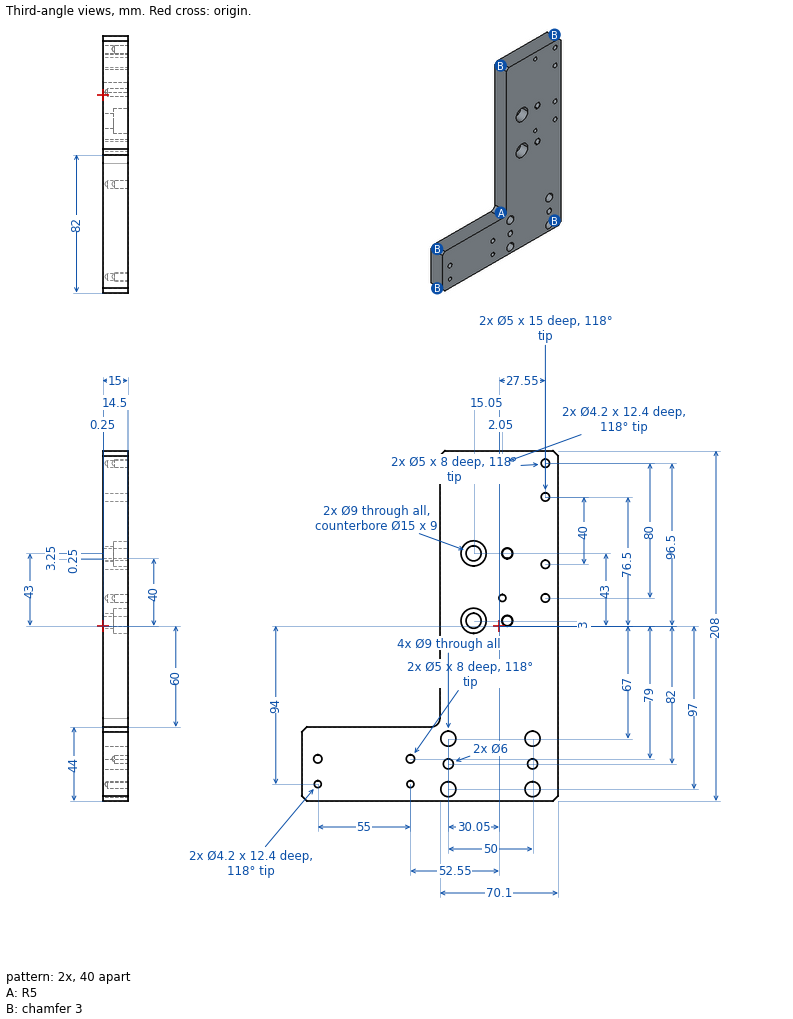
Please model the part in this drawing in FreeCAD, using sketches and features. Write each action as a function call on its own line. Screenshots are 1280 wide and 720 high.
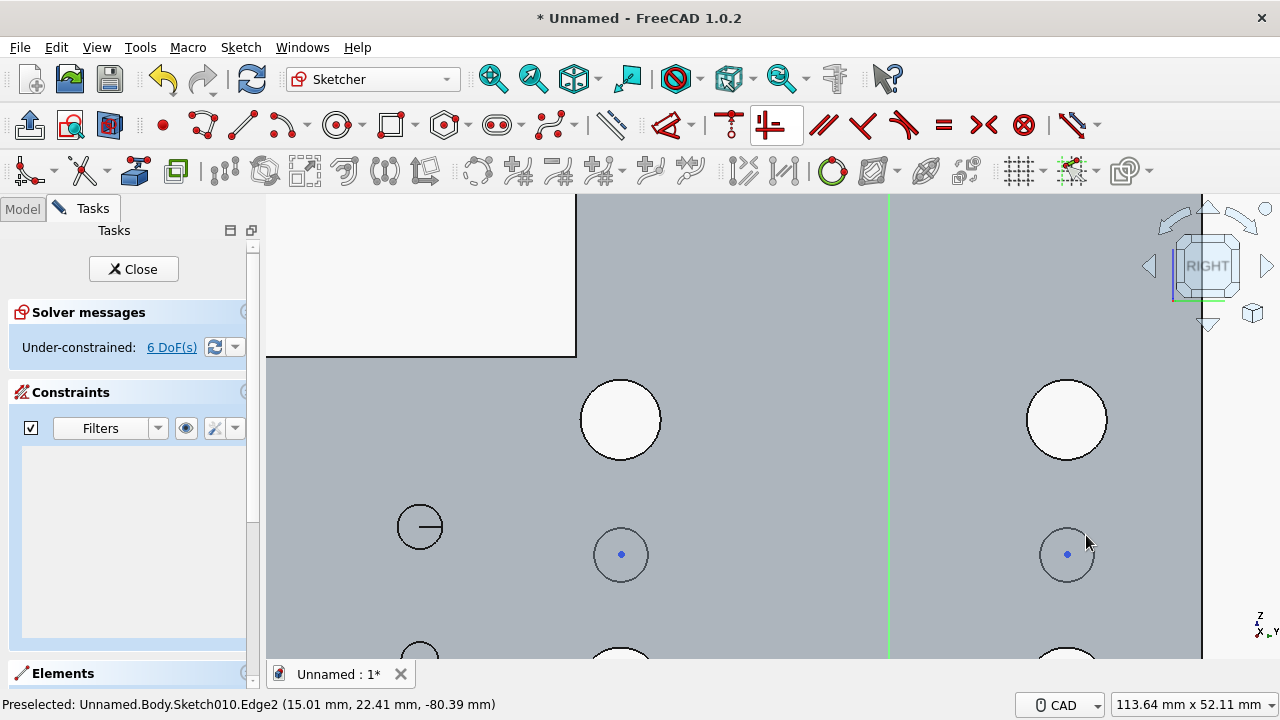
click(640, 536)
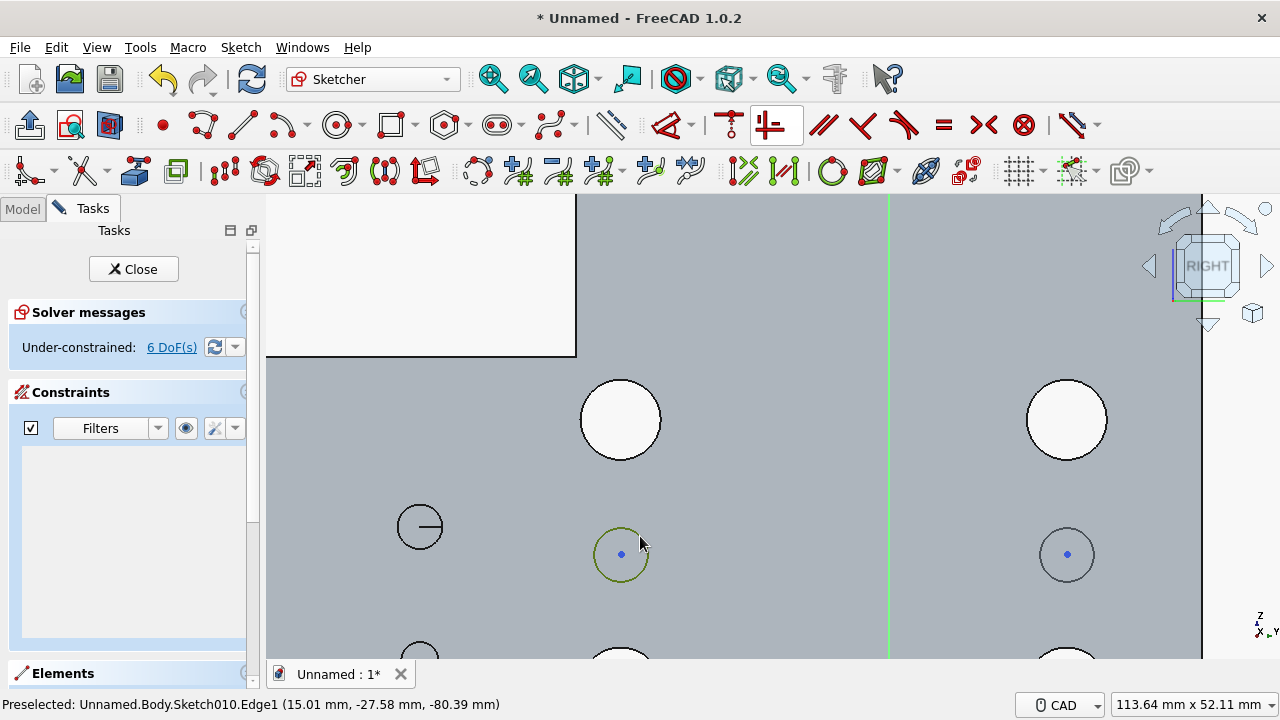
click(1086, 536)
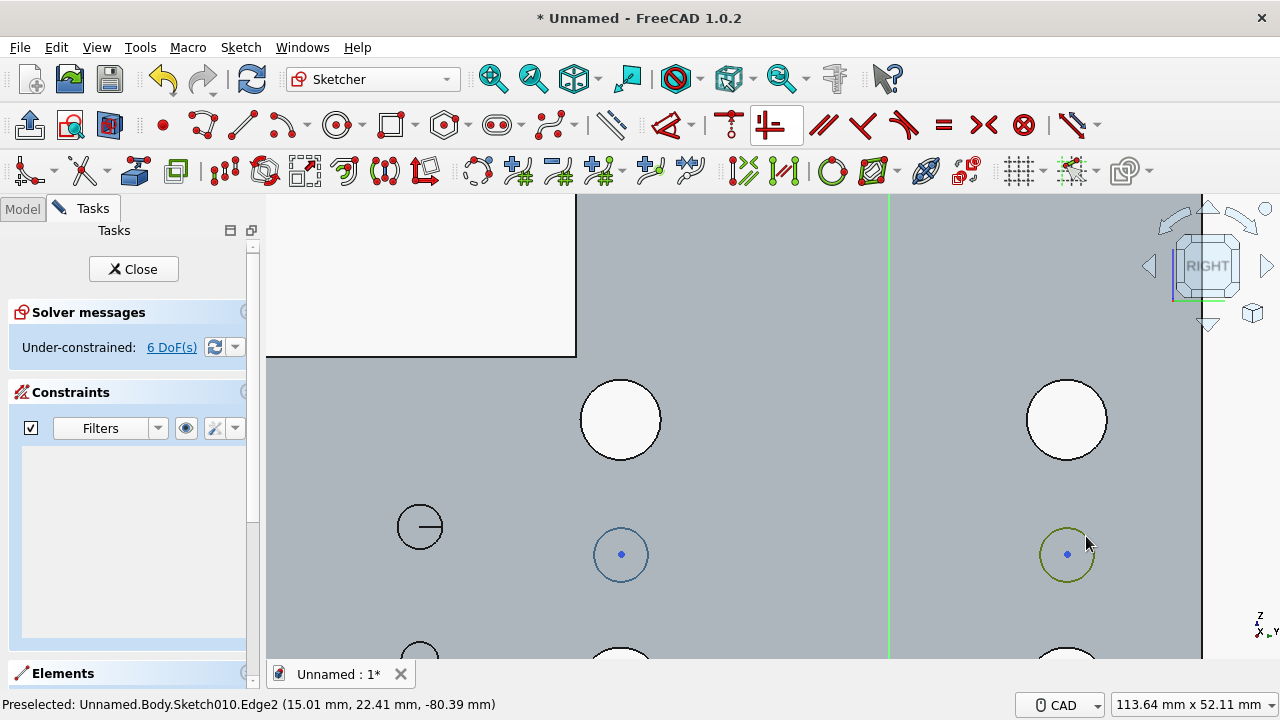
click(944, 126)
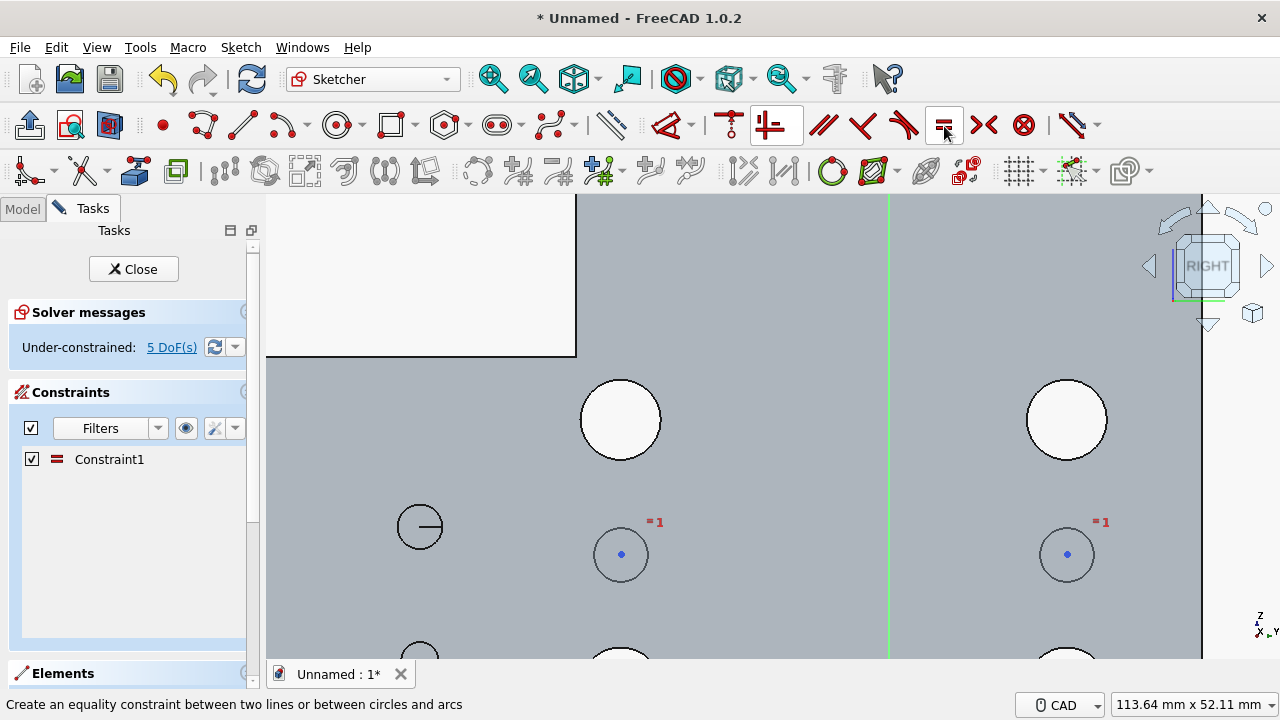
click(621, 555)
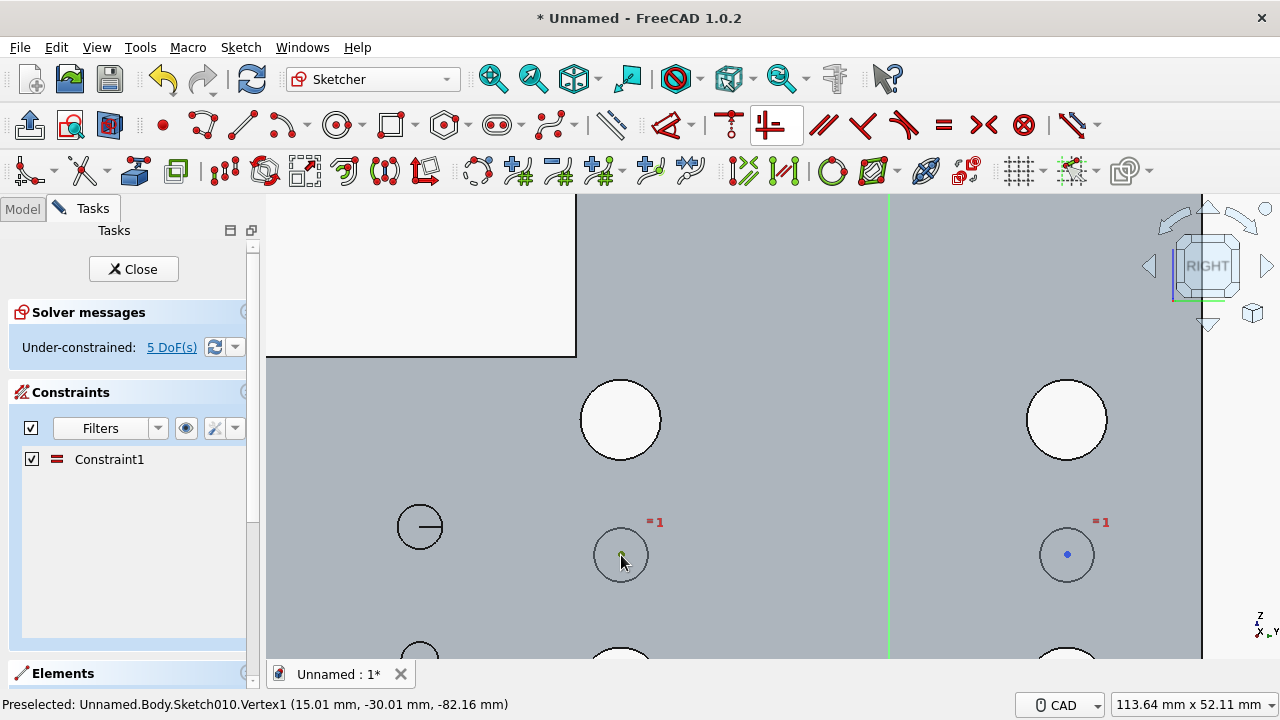
click(1067, 555)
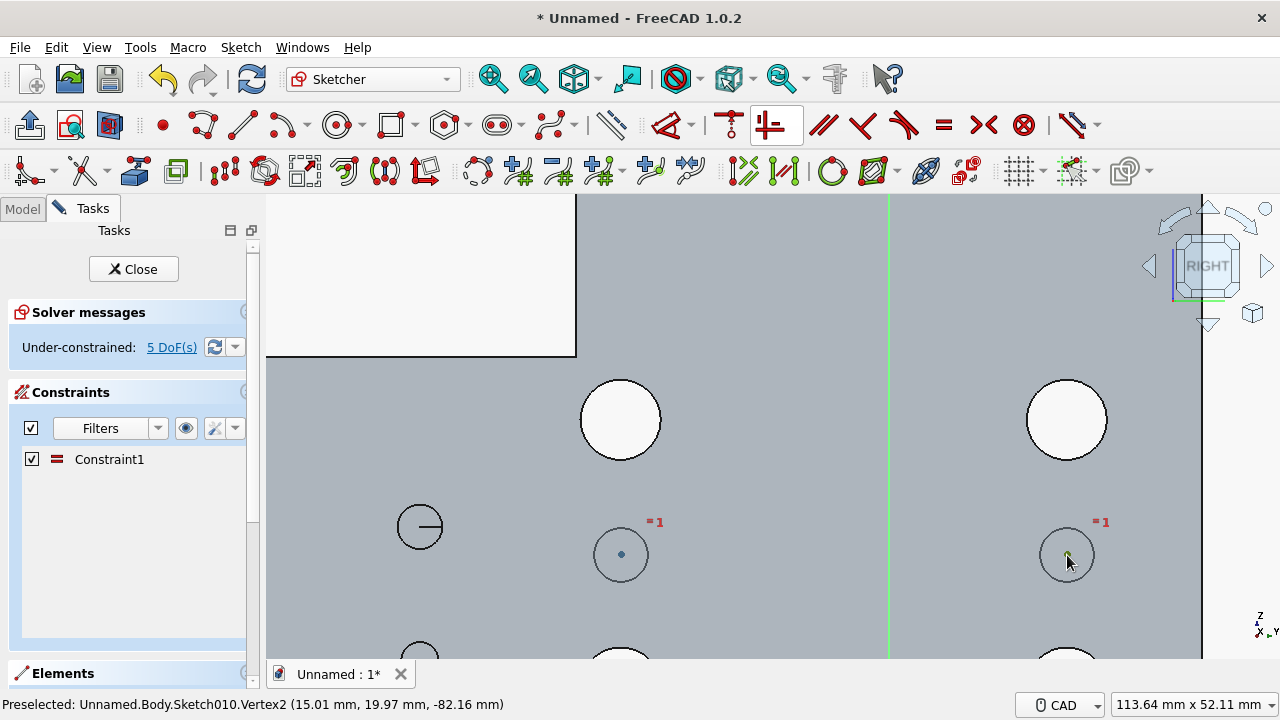
key(h)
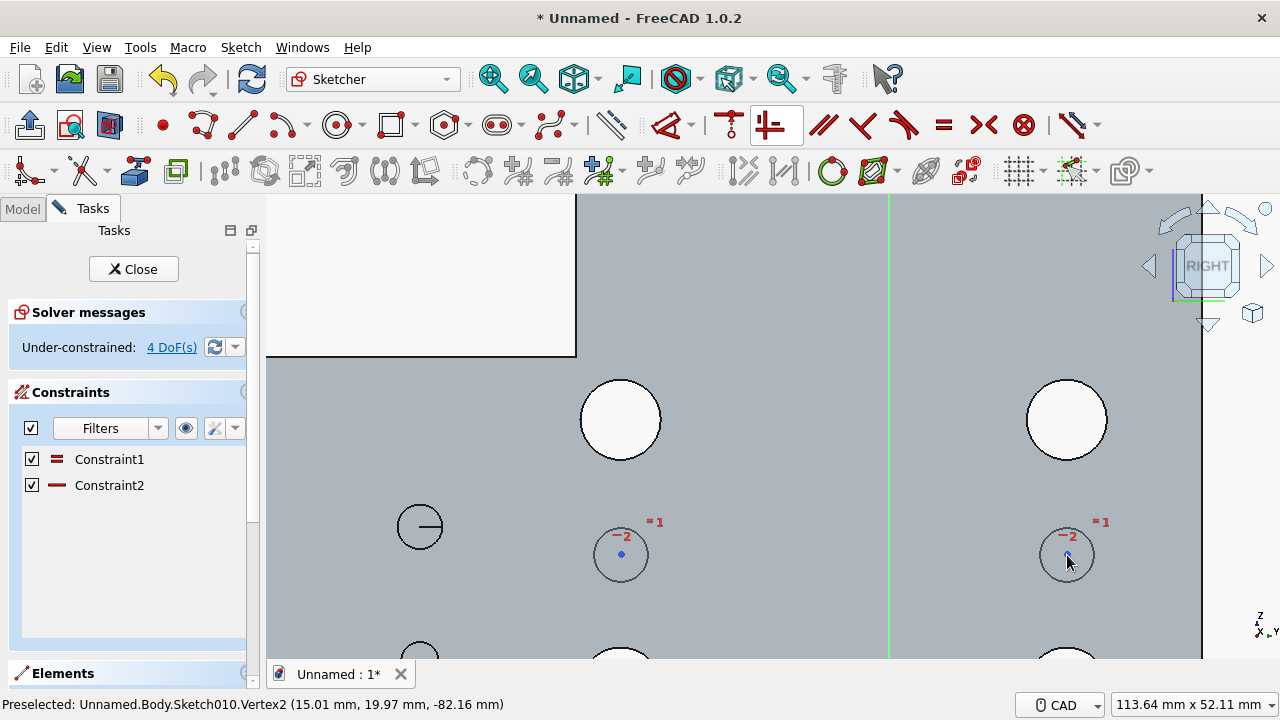
click(666, 126)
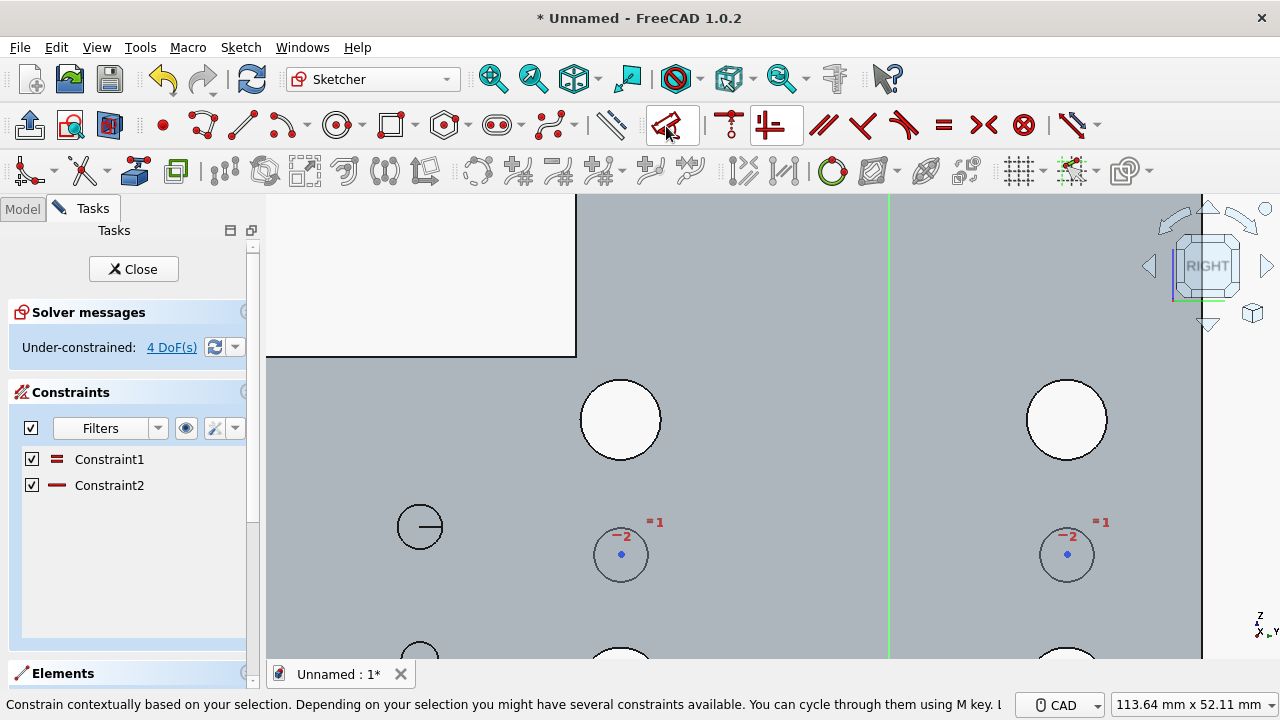
click(640, 536)
click(663, 513)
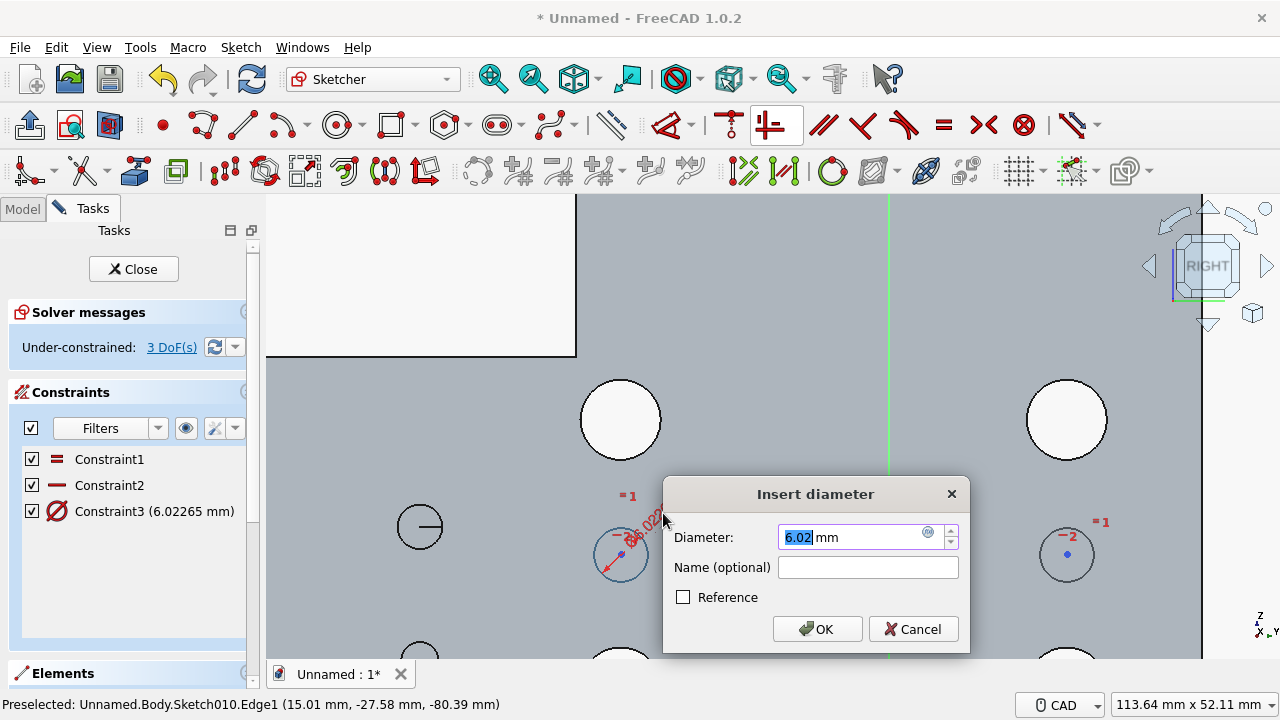
text(6)
key(Return)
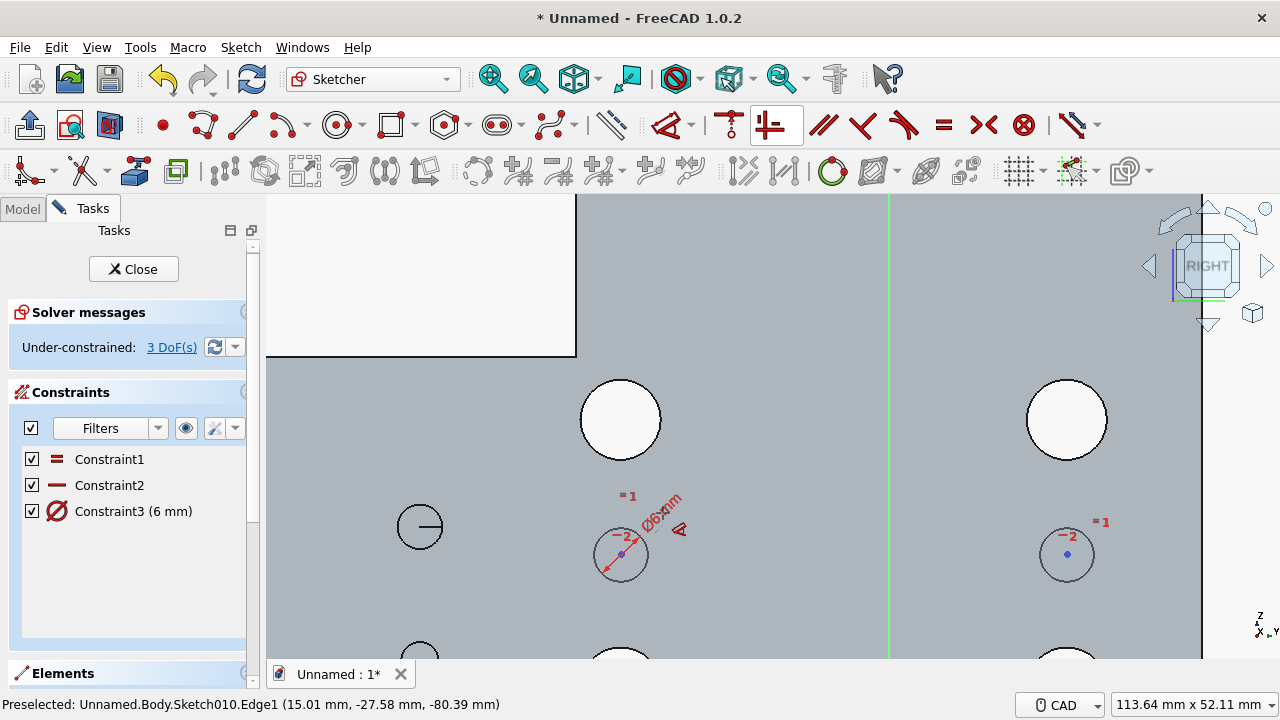
click(621, 555)
click(587, 388)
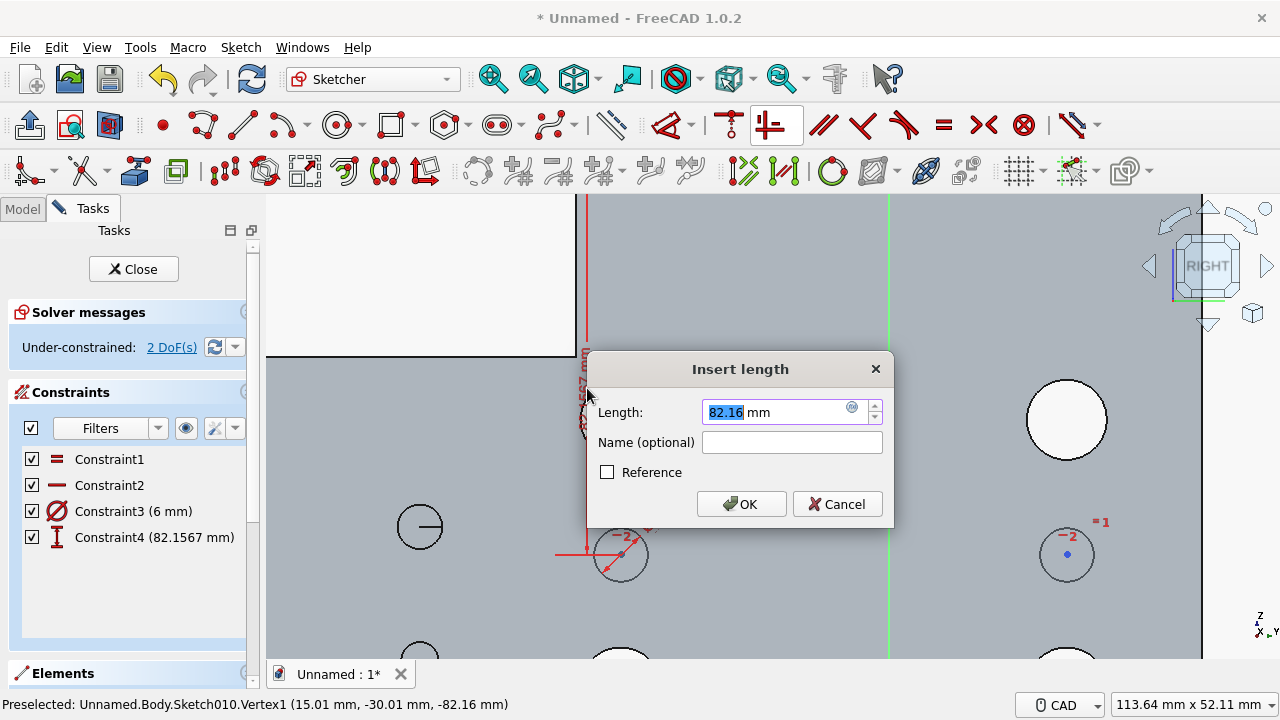
text(82)
key(Return)